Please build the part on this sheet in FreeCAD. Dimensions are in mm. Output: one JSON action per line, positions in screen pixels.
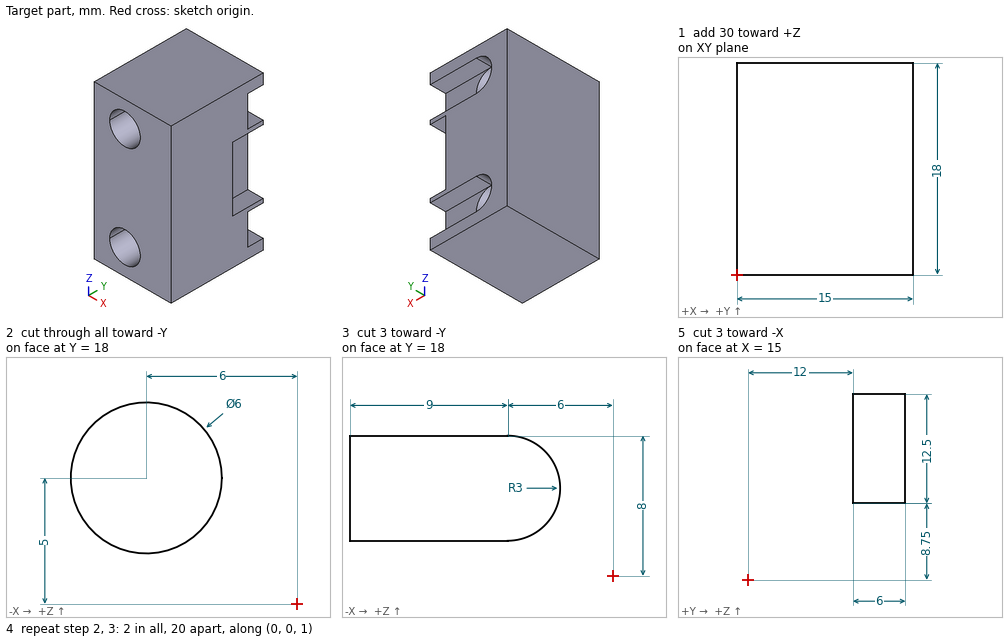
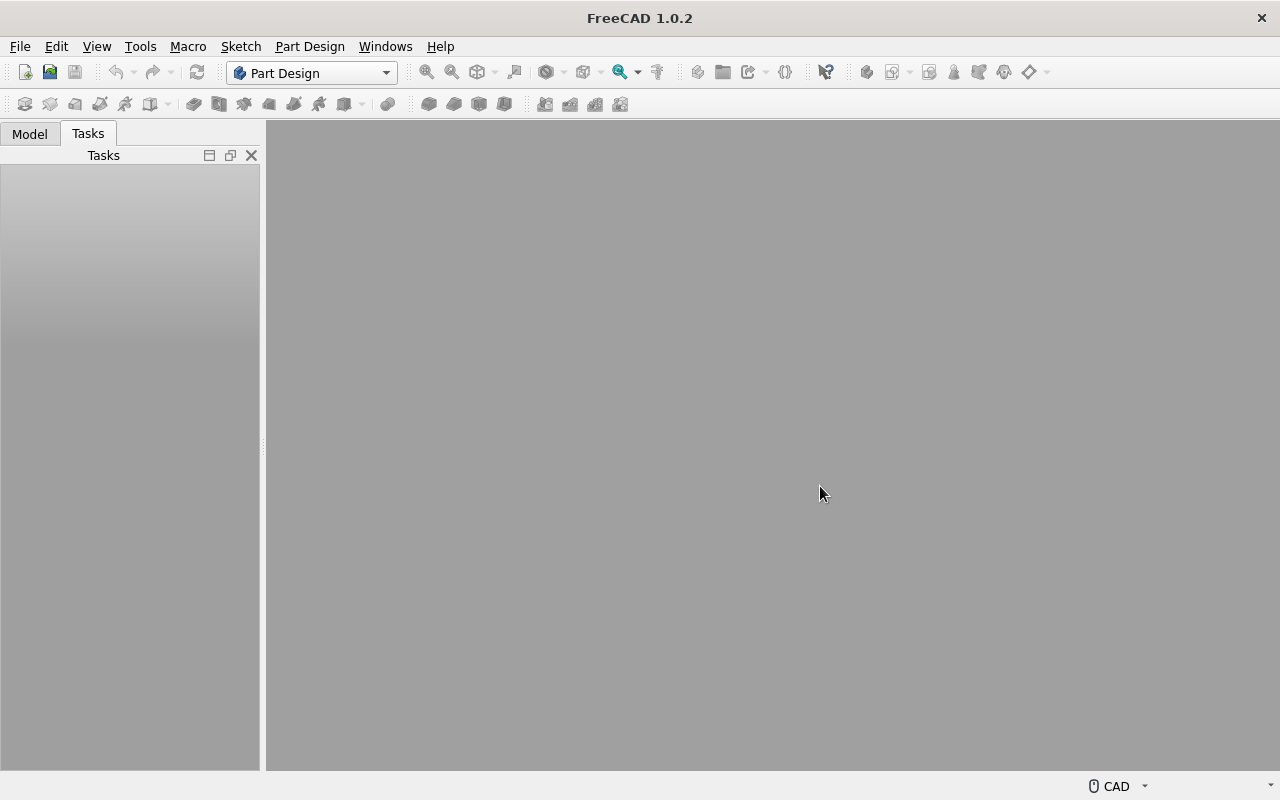
{"action": "left_click", "coordinate": [25, 72]}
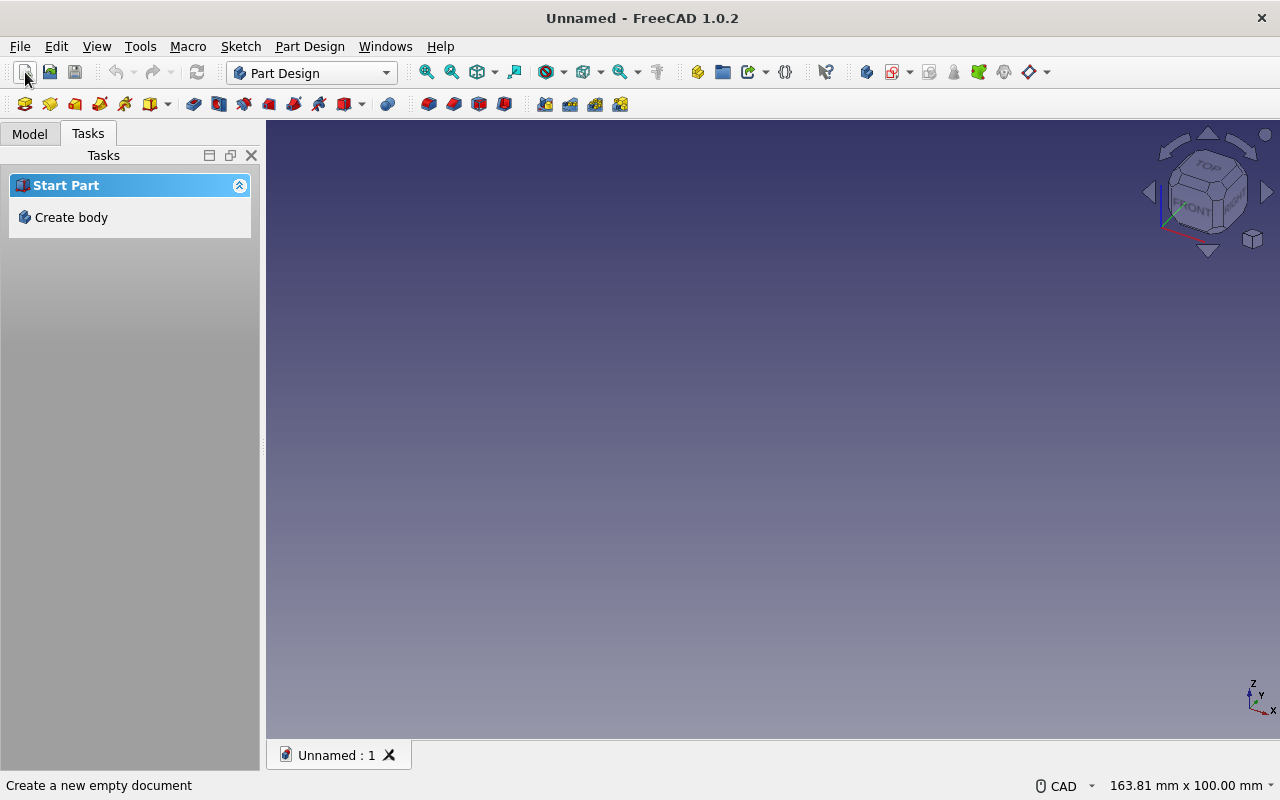
{"action": "left_click", "coordinate": [892, 72]}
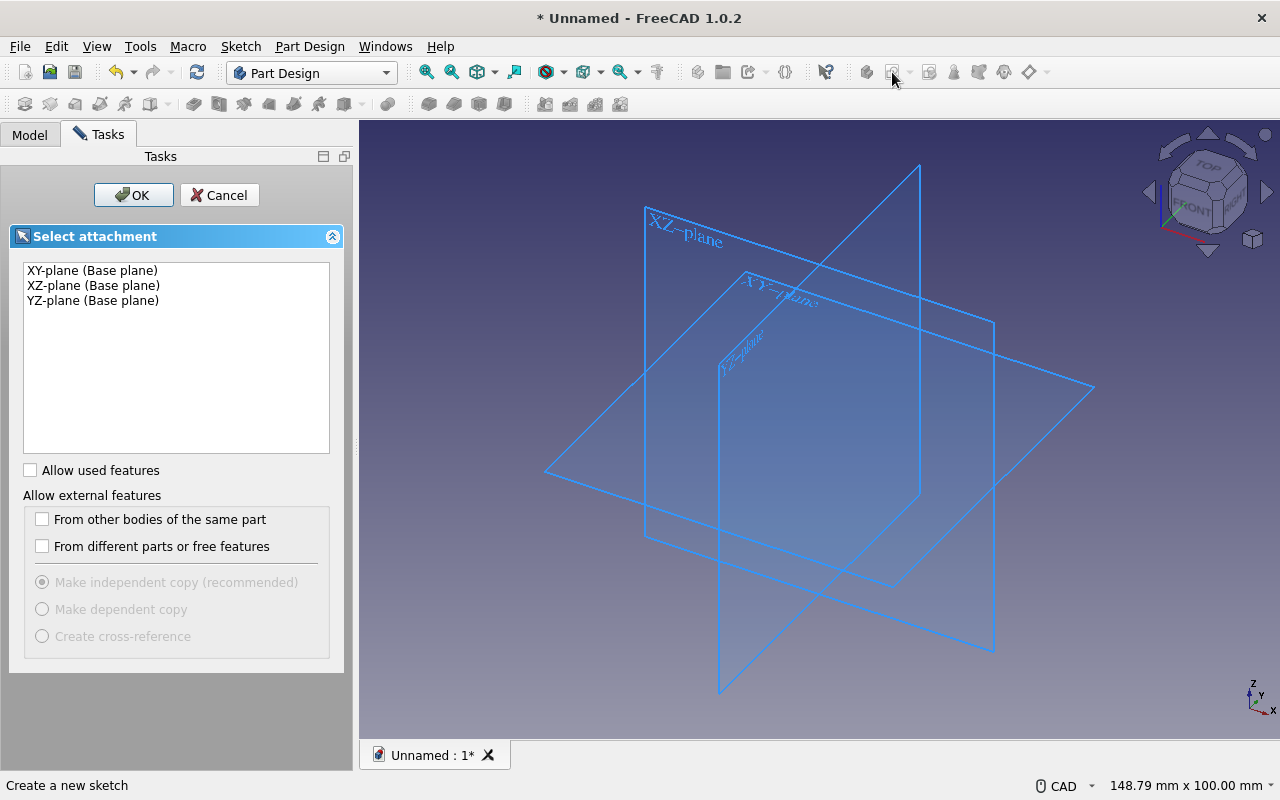
{"action": "left_click", "coordinate": [84, 270]}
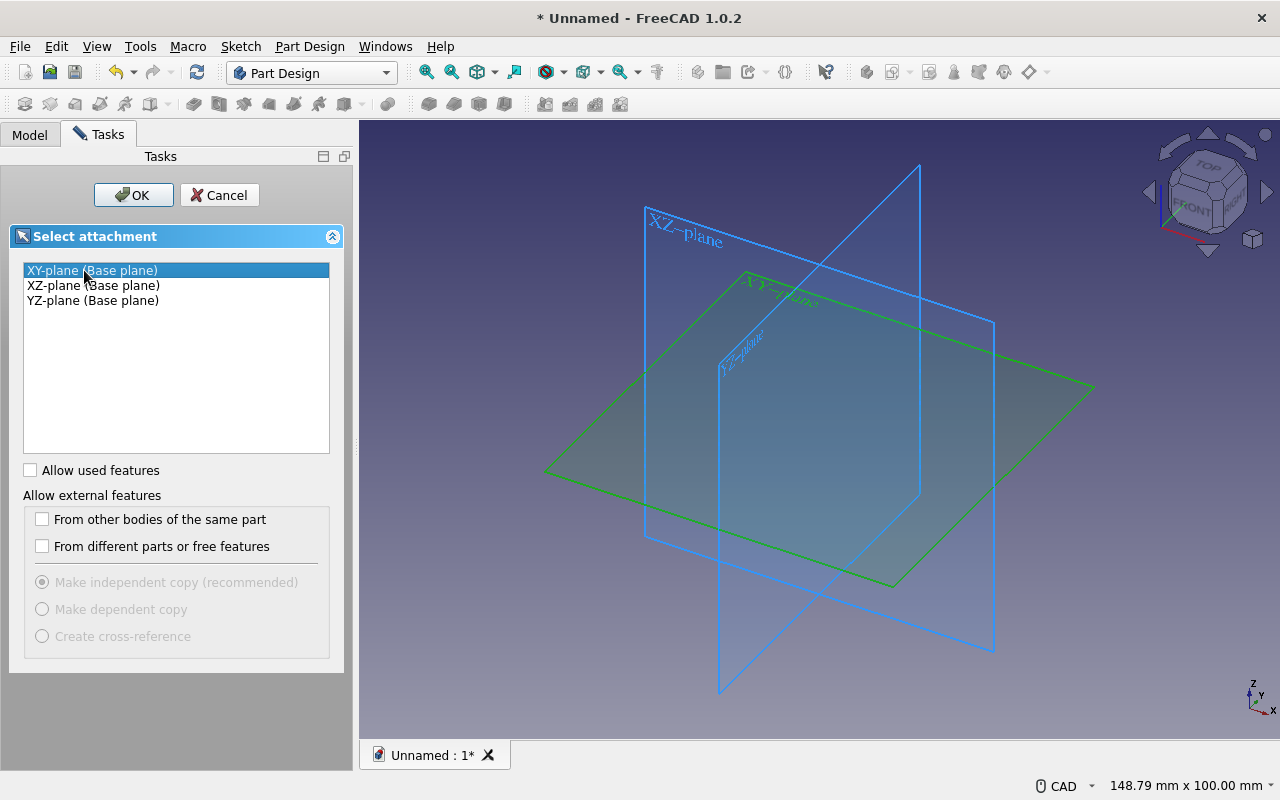
{"action": "left_click", "coordinate": [134, 195]}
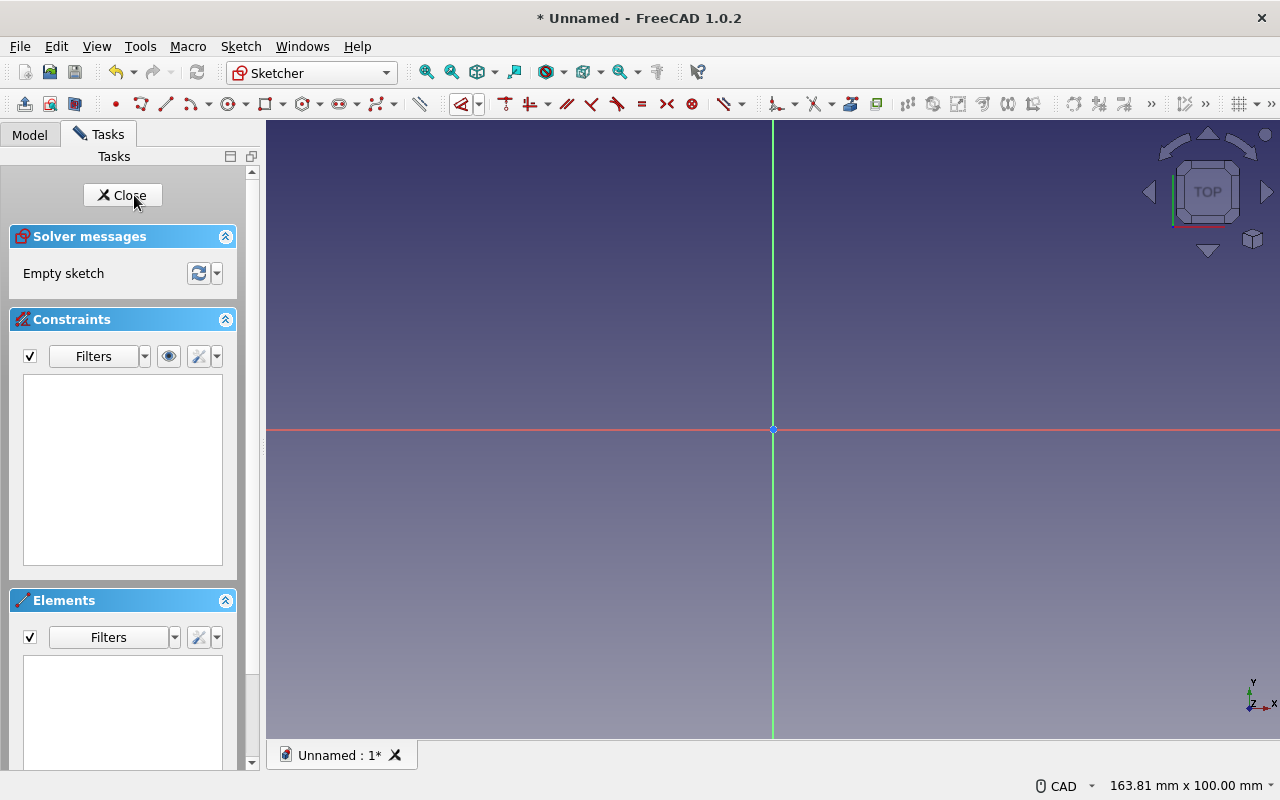
{"action": "scroll", "coordinate": [869, 350], "scroll_direction": "up", "scroll_amount": 6}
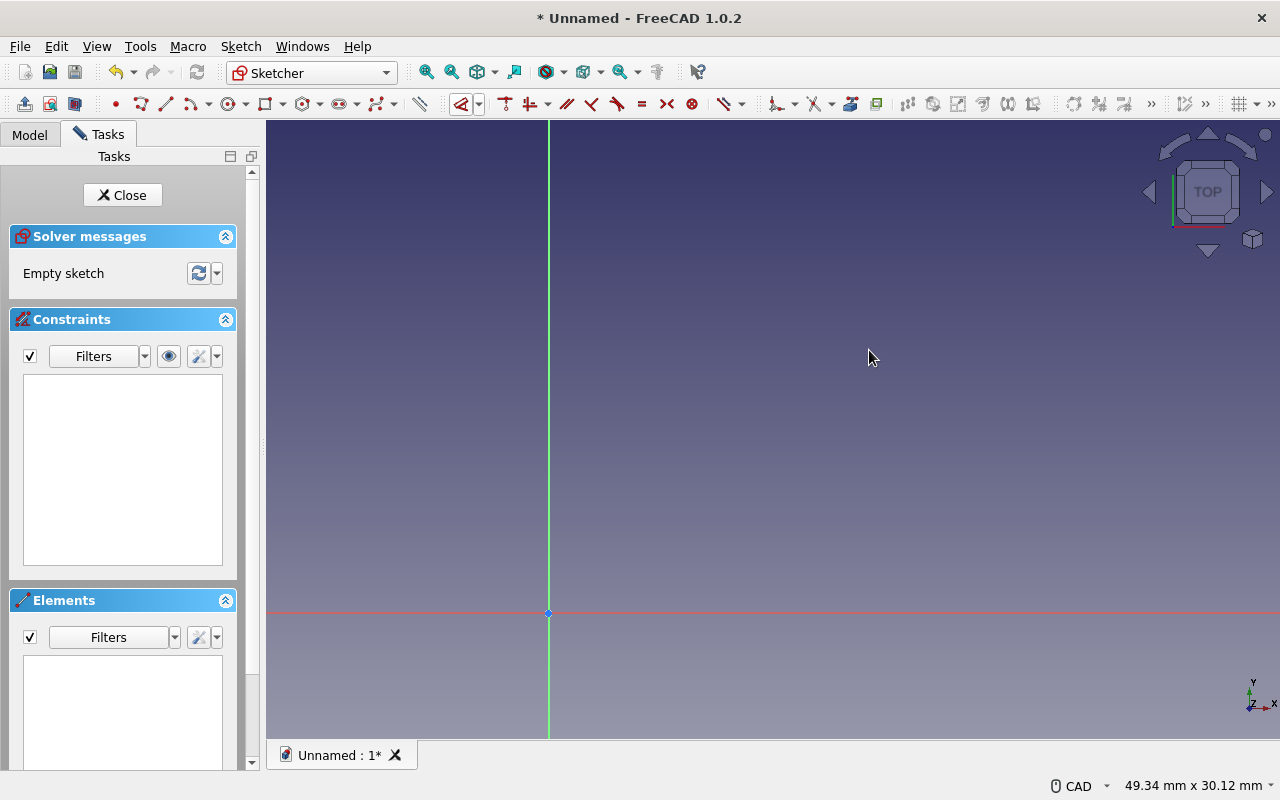
{"action": "left_click", "coordinate": [264, 104]}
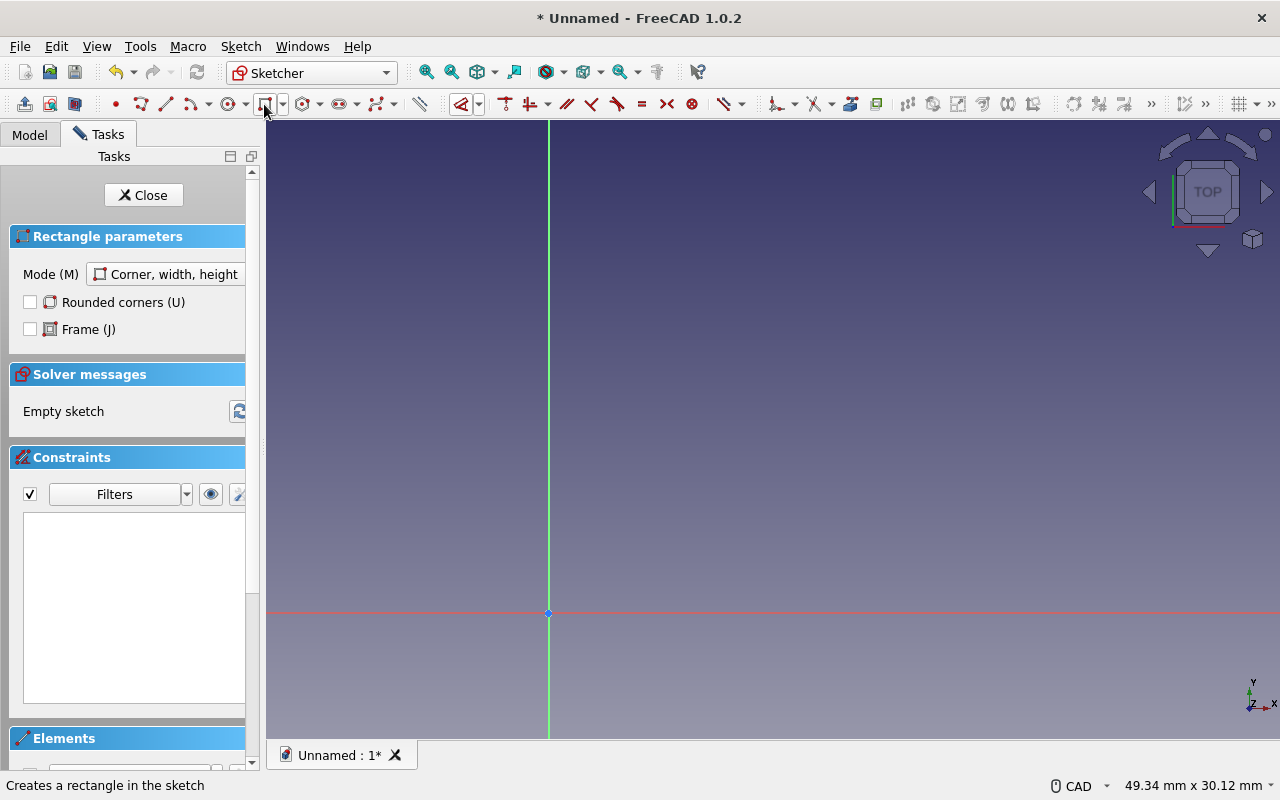
{"action": "left_click", "coordinate": [549, 613]}
{"action": "mouse_move", "coordinate": [857, 243]}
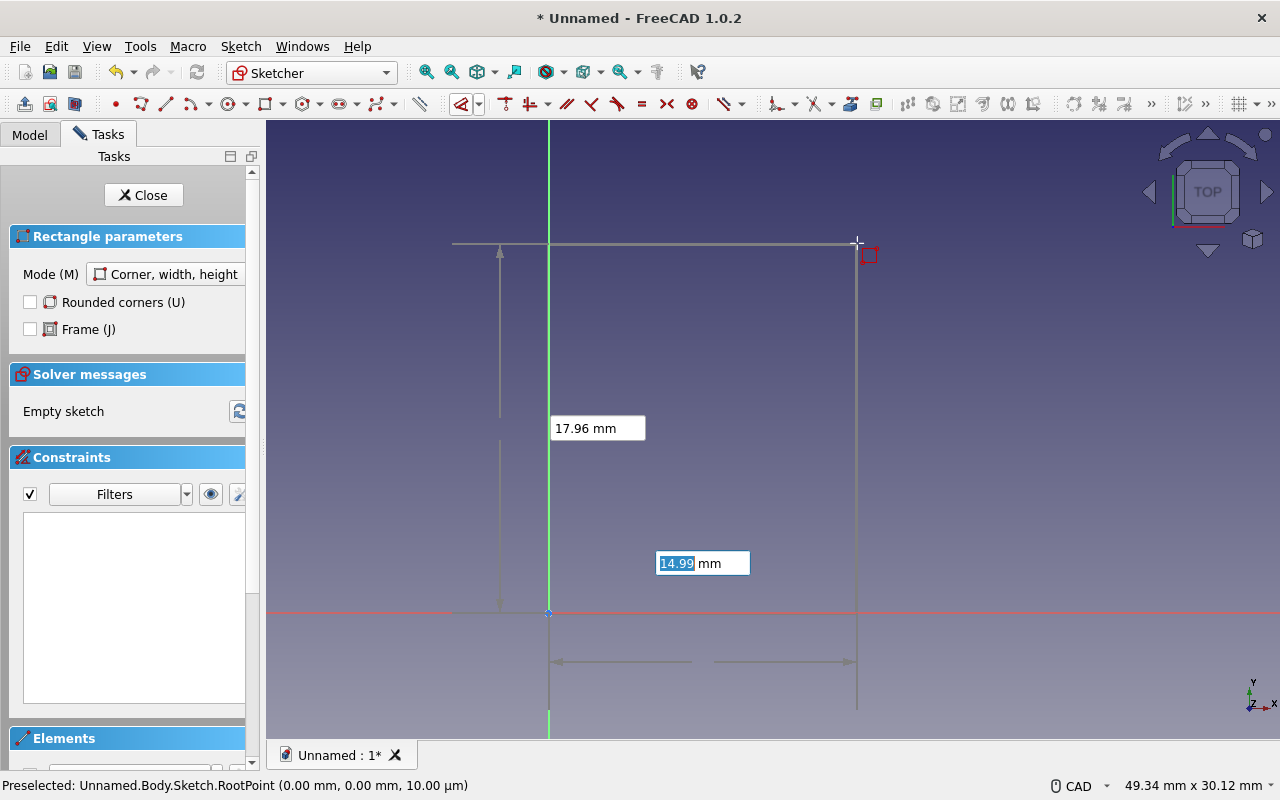
{"action": "type", "text": "15"}
{"action": "key", "text": "Tab"}
{"action": "type", "text": "18"}
{"action": "key", "text": "Return"}
{"action": "key", "text": "Escape"}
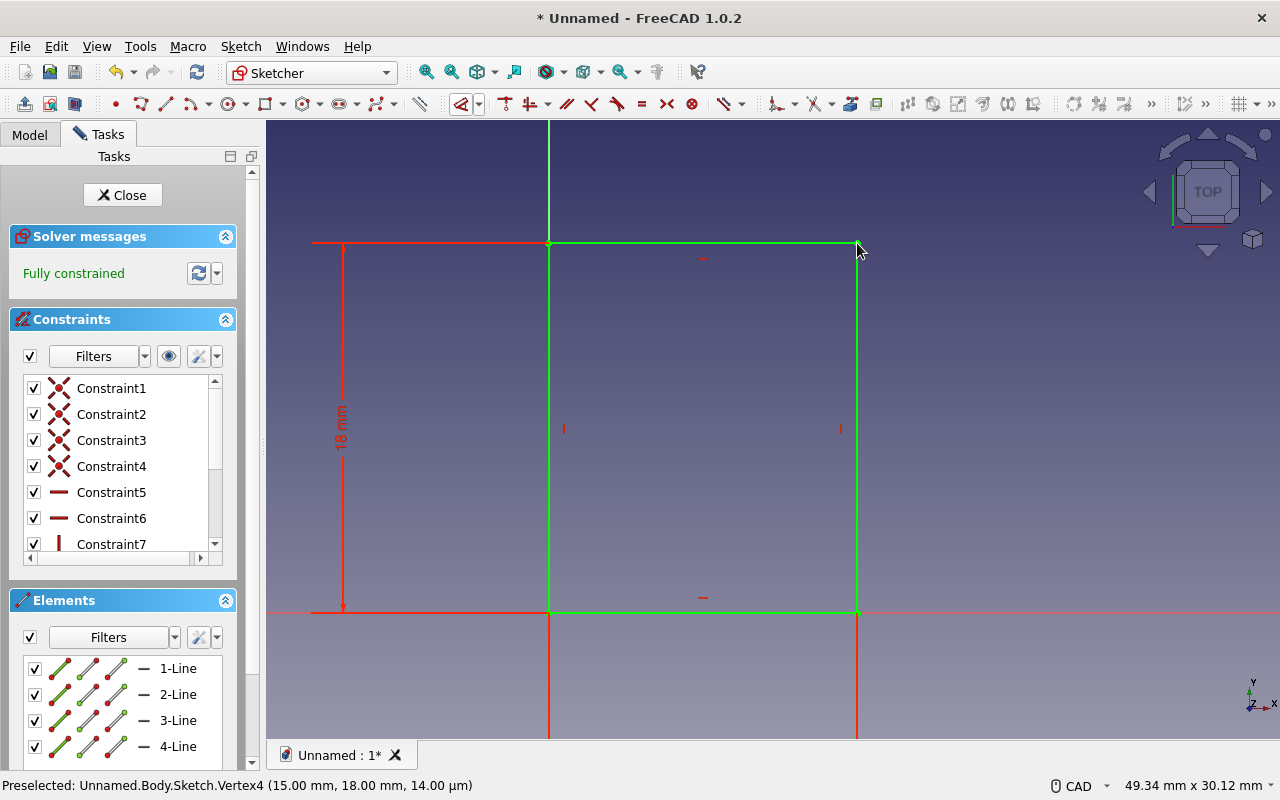
{"action": "left_click", "coordinate": [123, 195]}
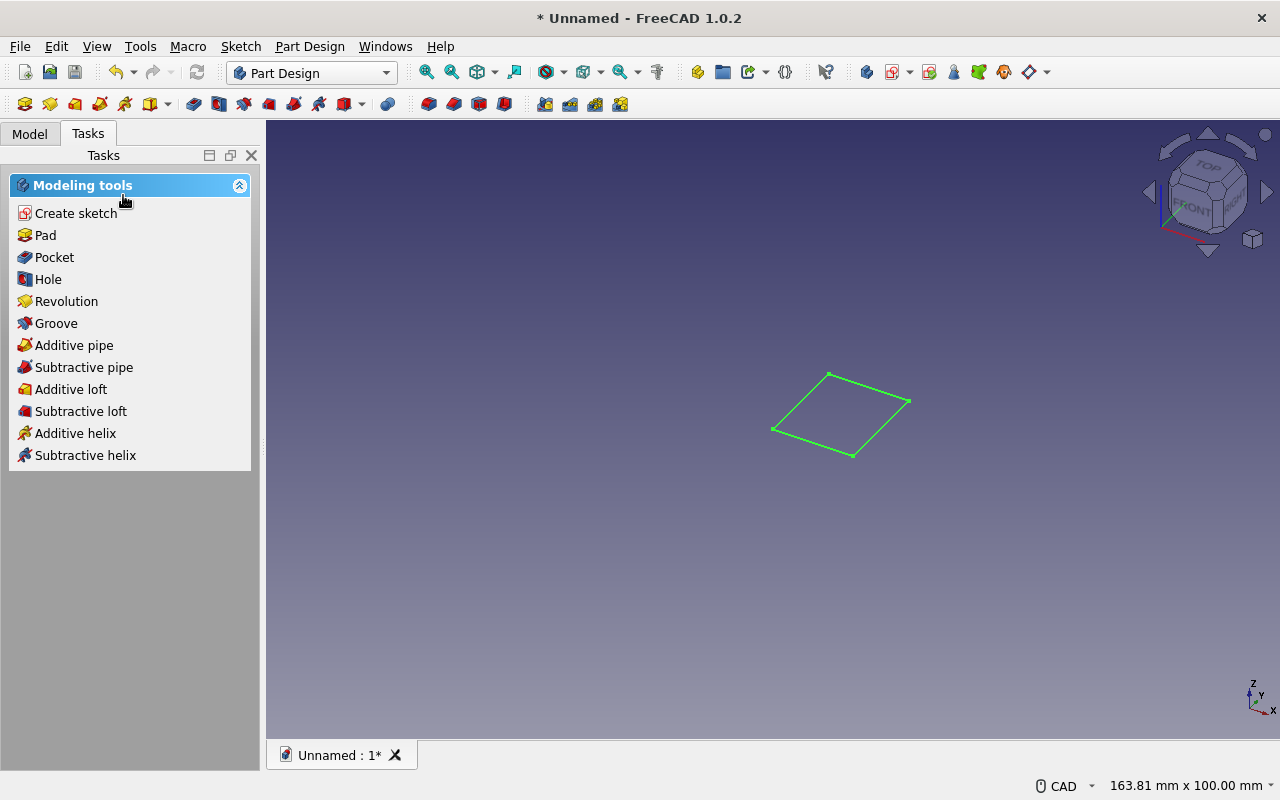
{"action": "left_click", "coordinate": [25, 104]}